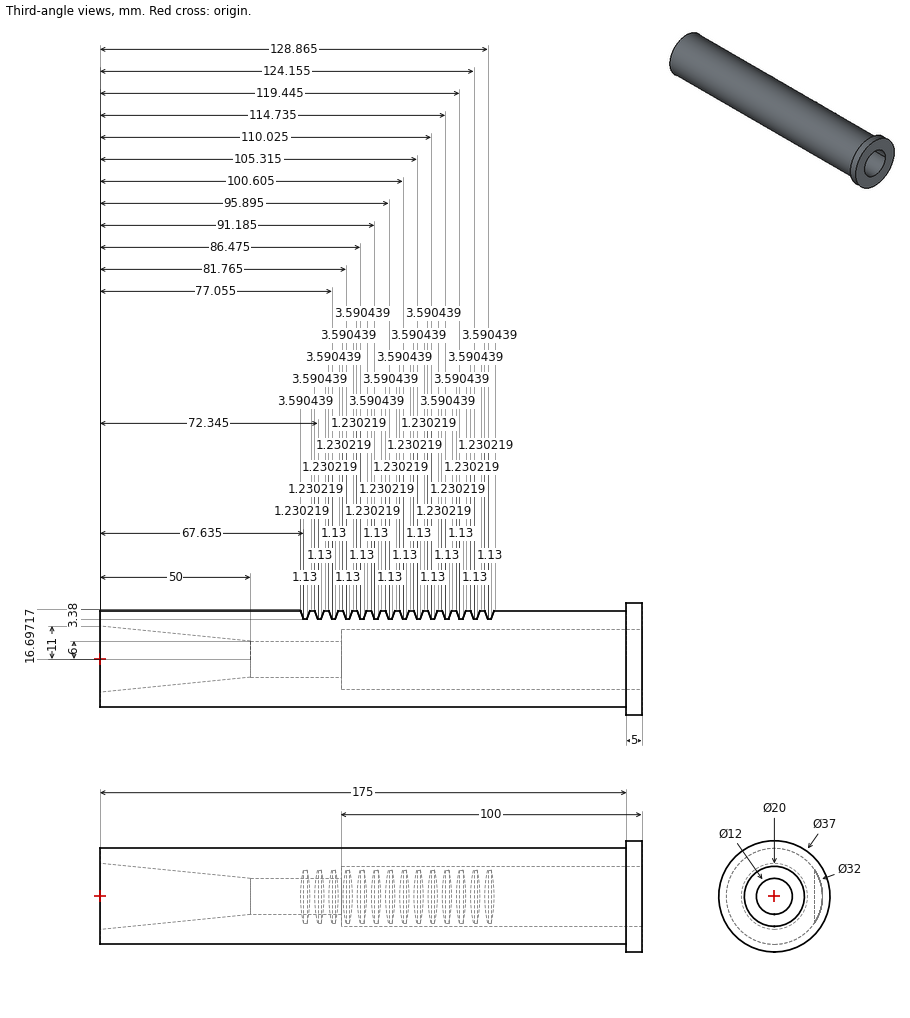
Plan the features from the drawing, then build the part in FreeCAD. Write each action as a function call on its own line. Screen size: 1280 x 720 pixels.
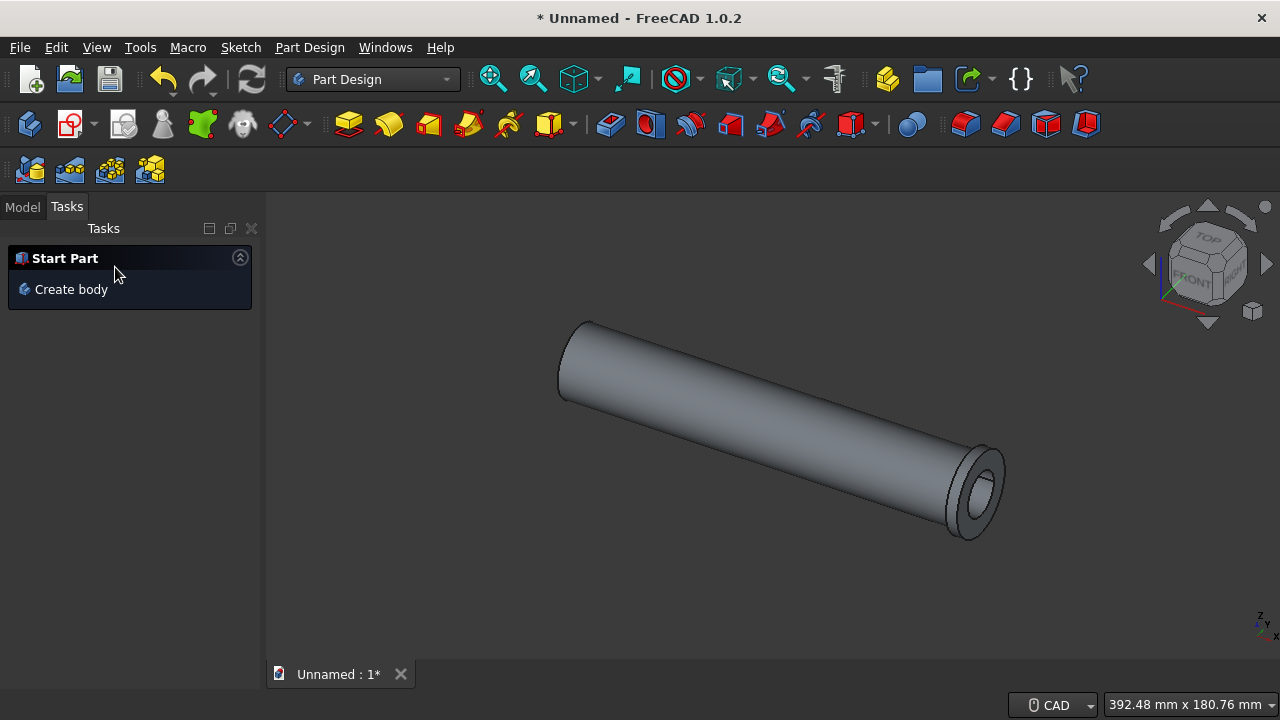
click(995, 457)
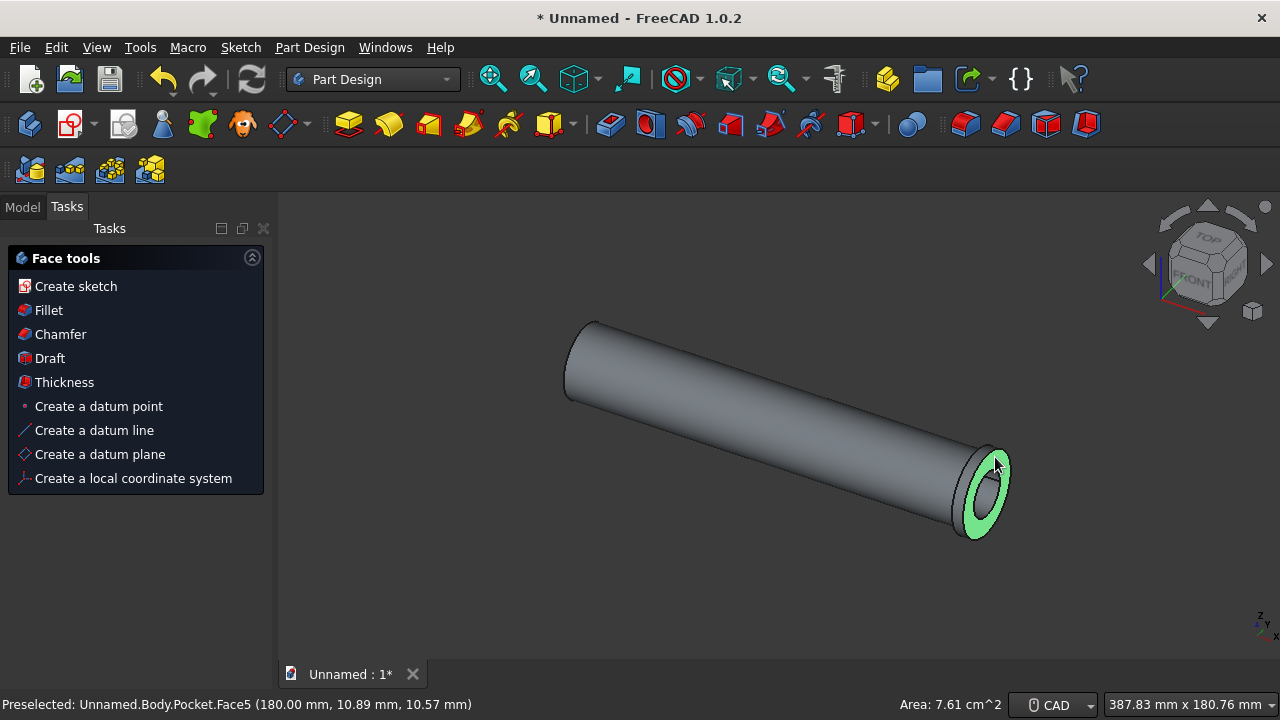
click(70, 124)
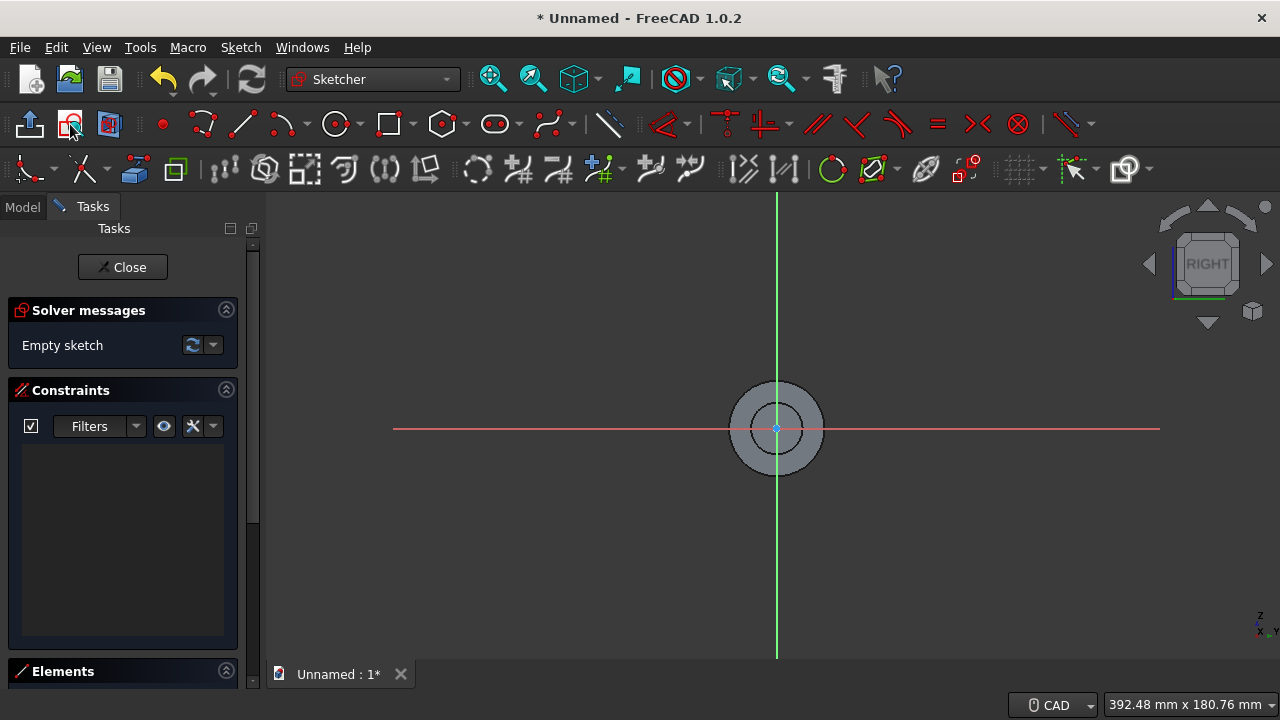
scroll(786, 429, up, 11)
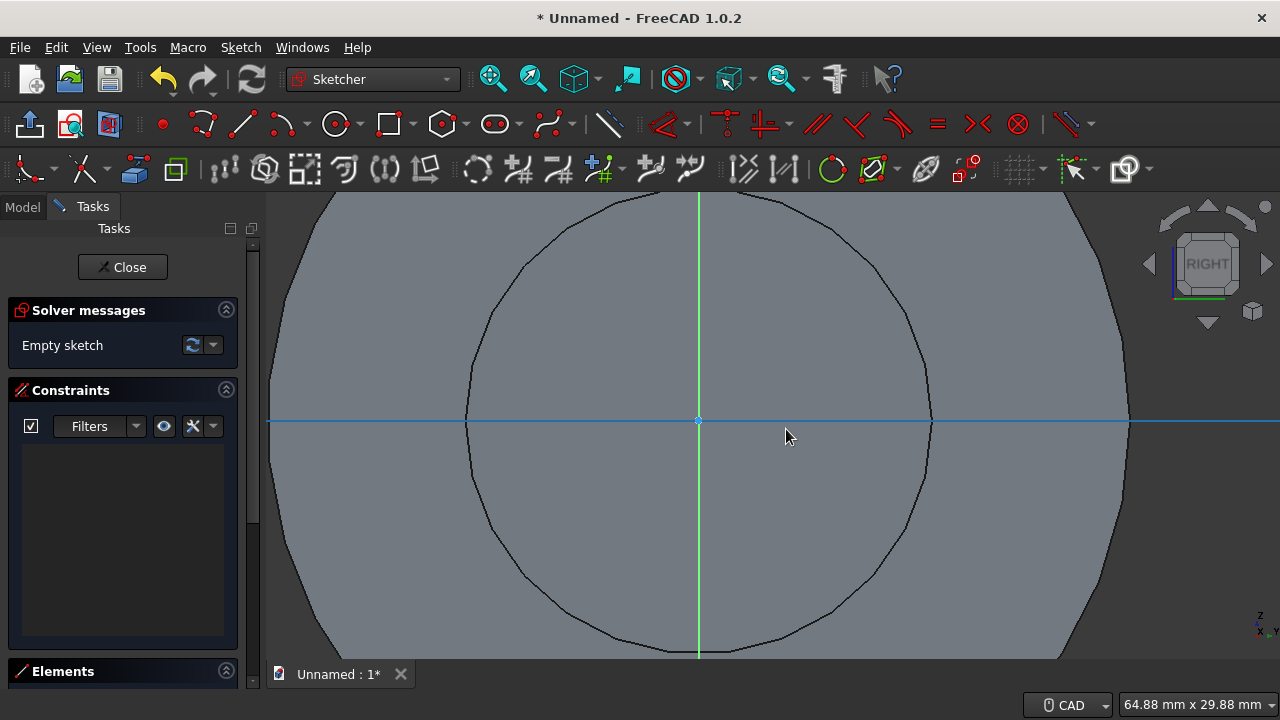
key(g)
key(c)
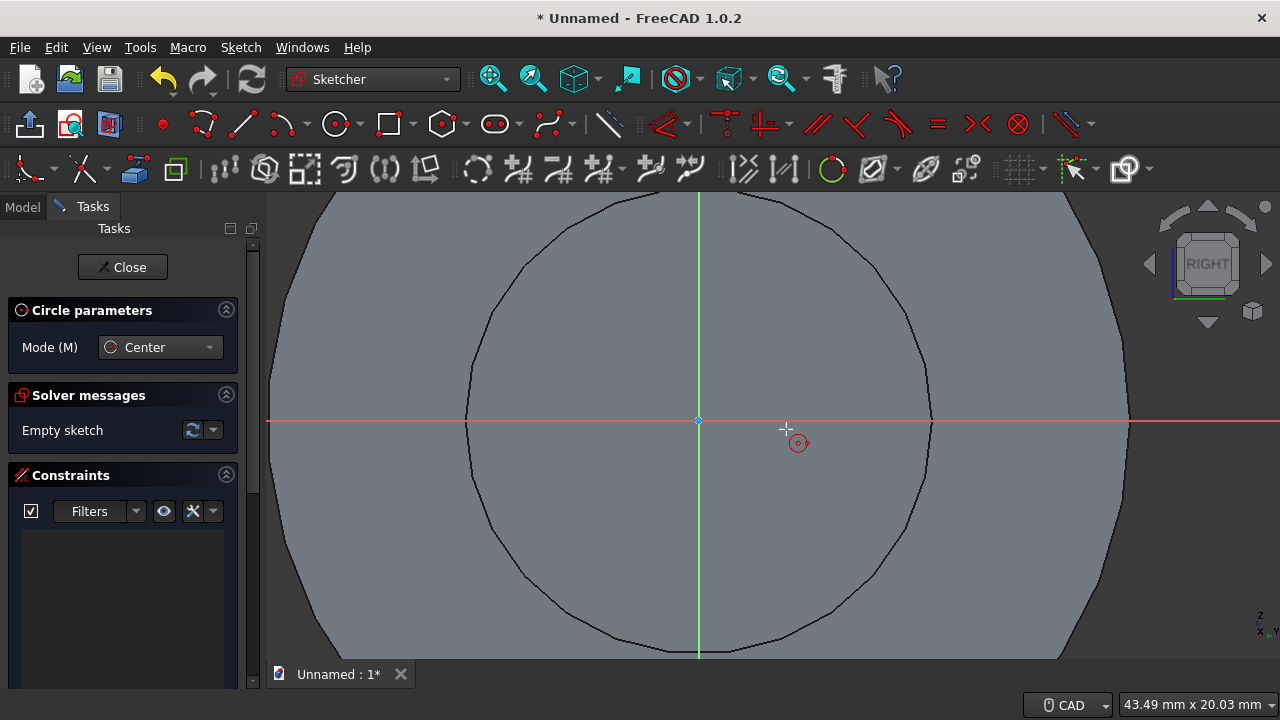
click(699, 421)
move(798, 322)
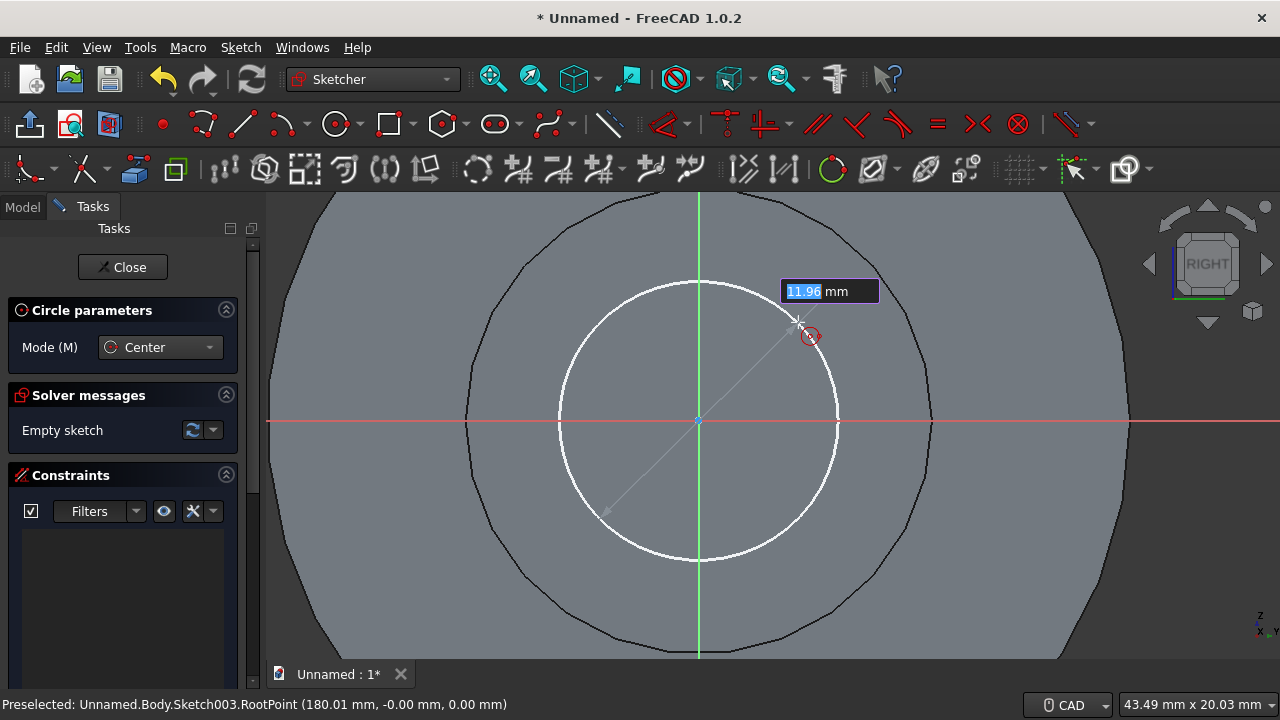
text(12)
key(Return)
key(Escape)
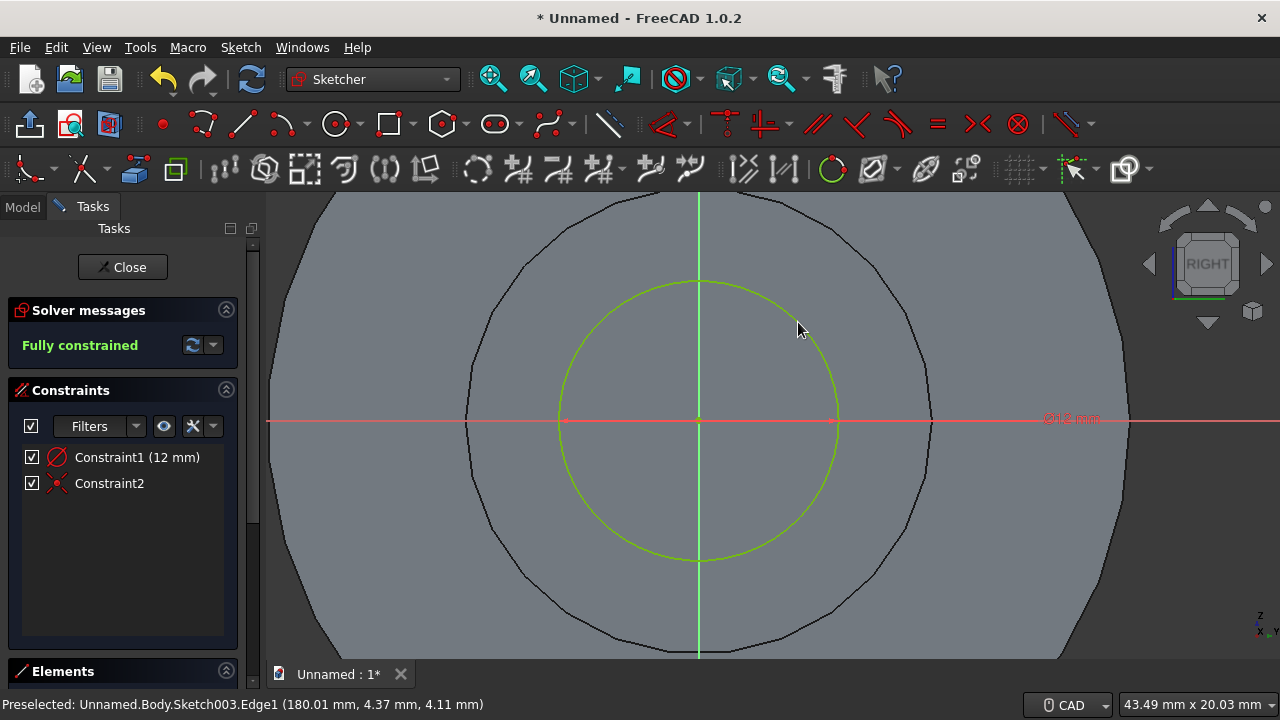
click(123, 267)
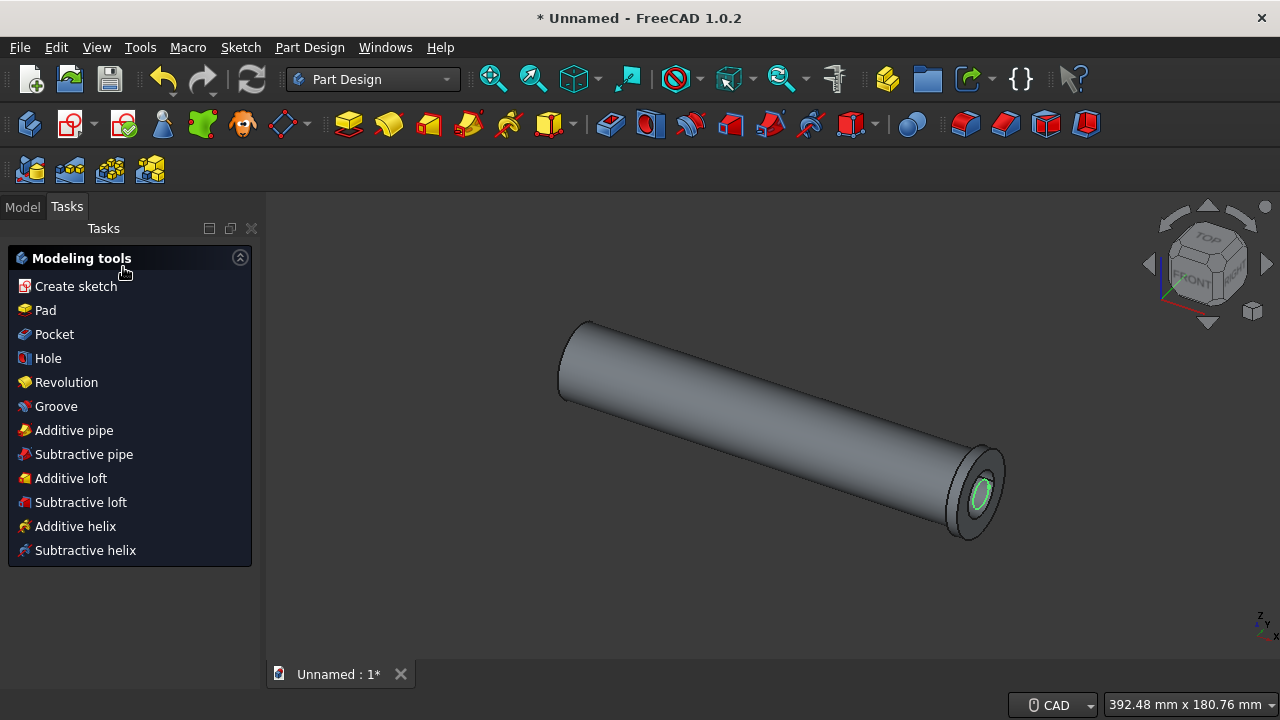
click(612, 124)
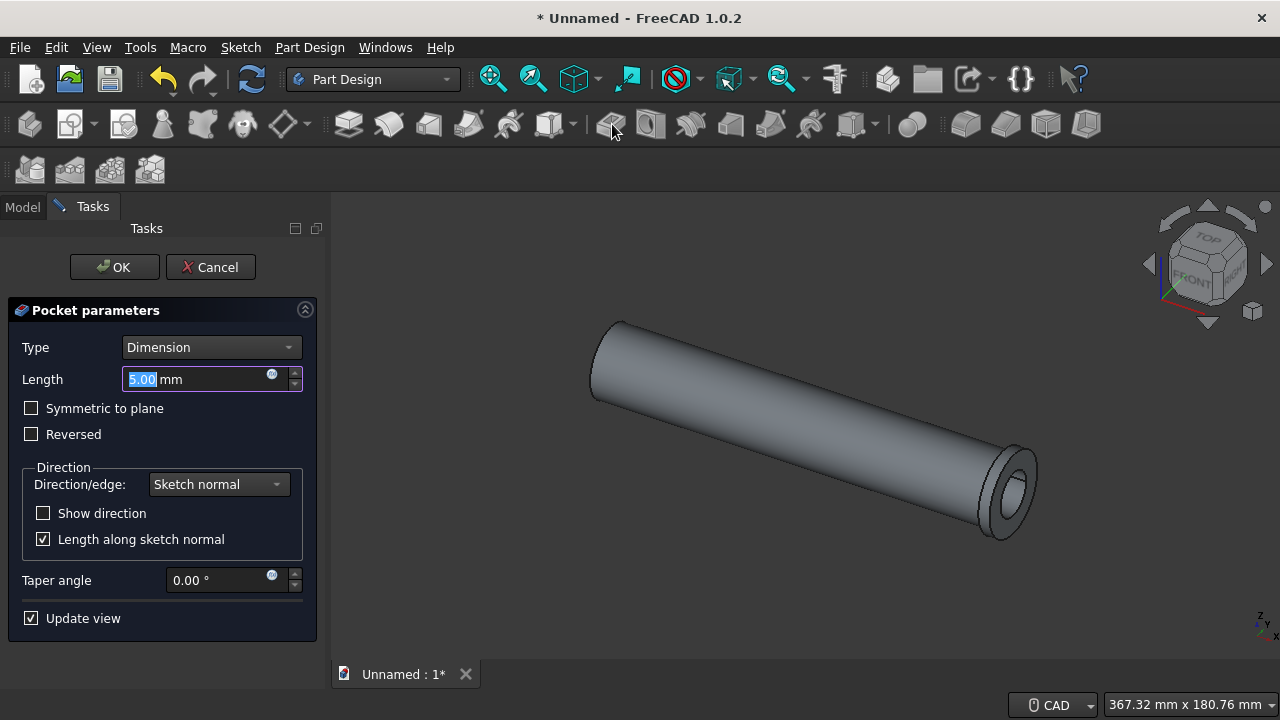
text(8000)
key(Tab)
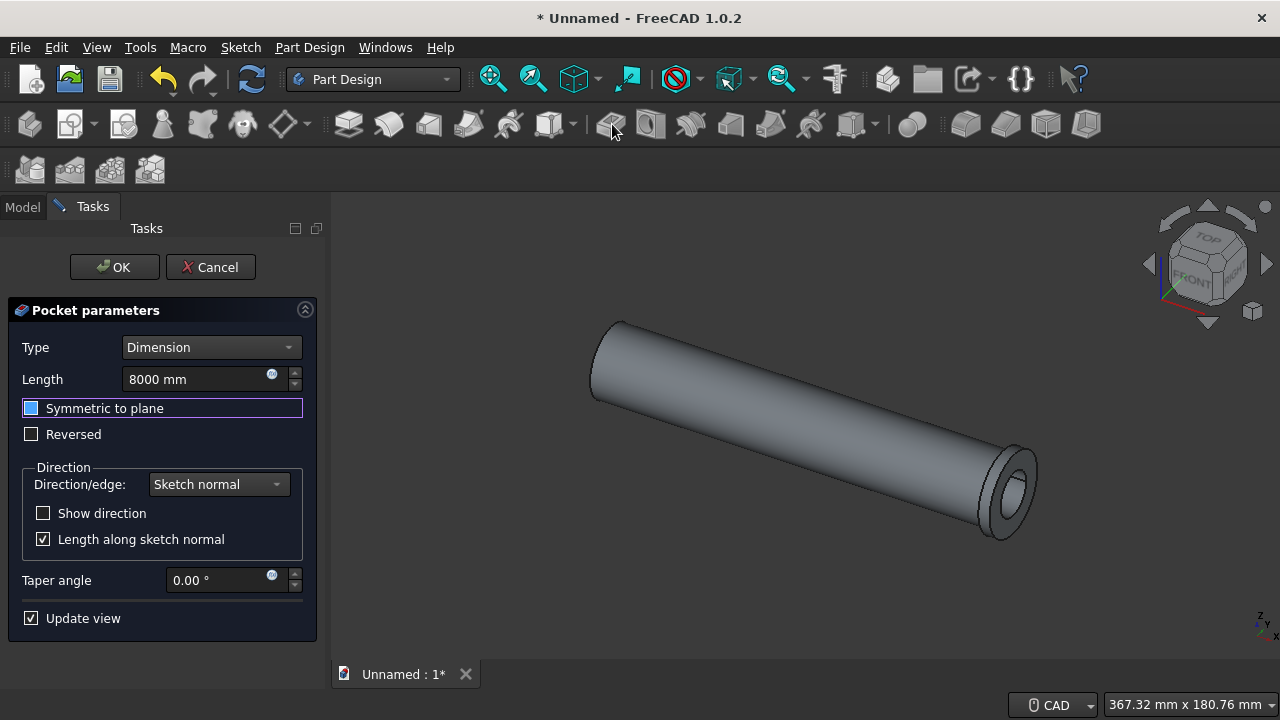
click(115, 267)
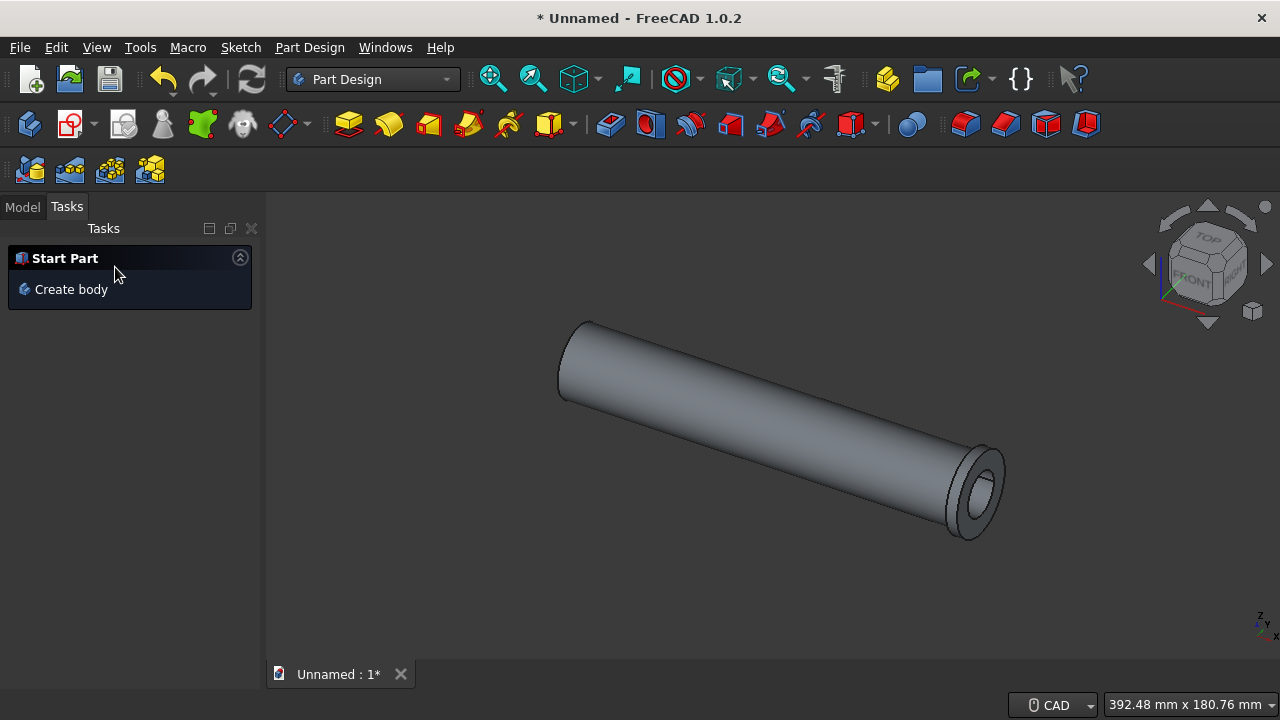
click(70, 124)